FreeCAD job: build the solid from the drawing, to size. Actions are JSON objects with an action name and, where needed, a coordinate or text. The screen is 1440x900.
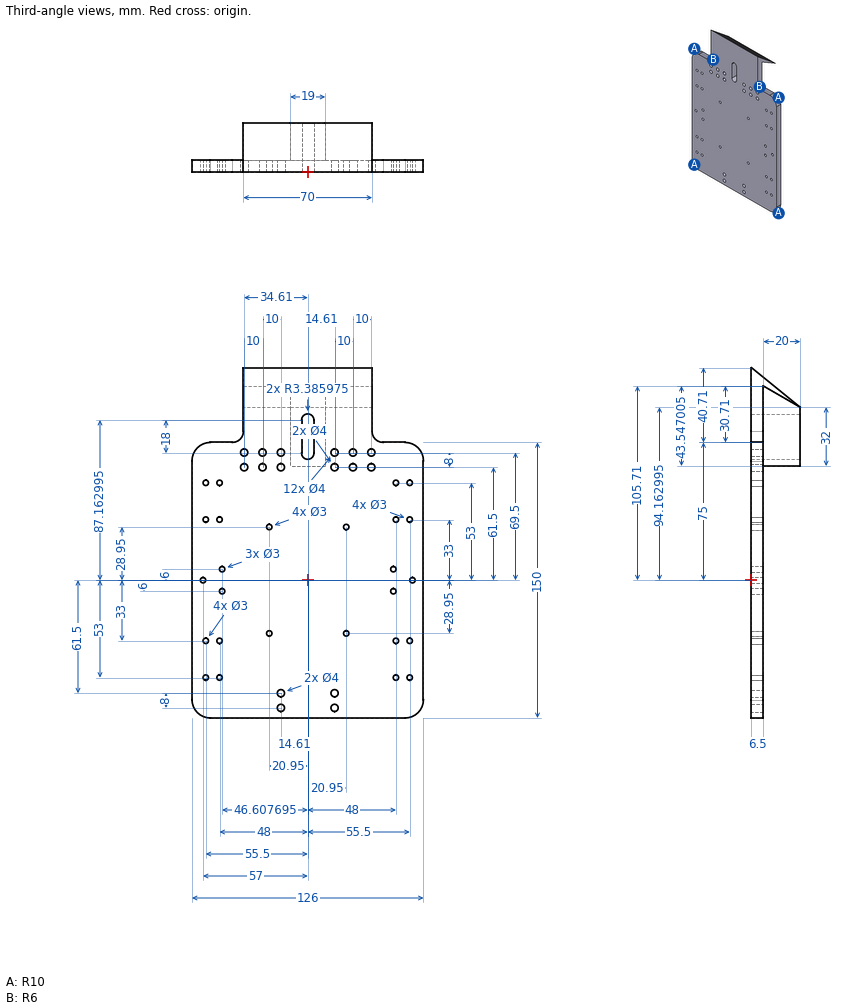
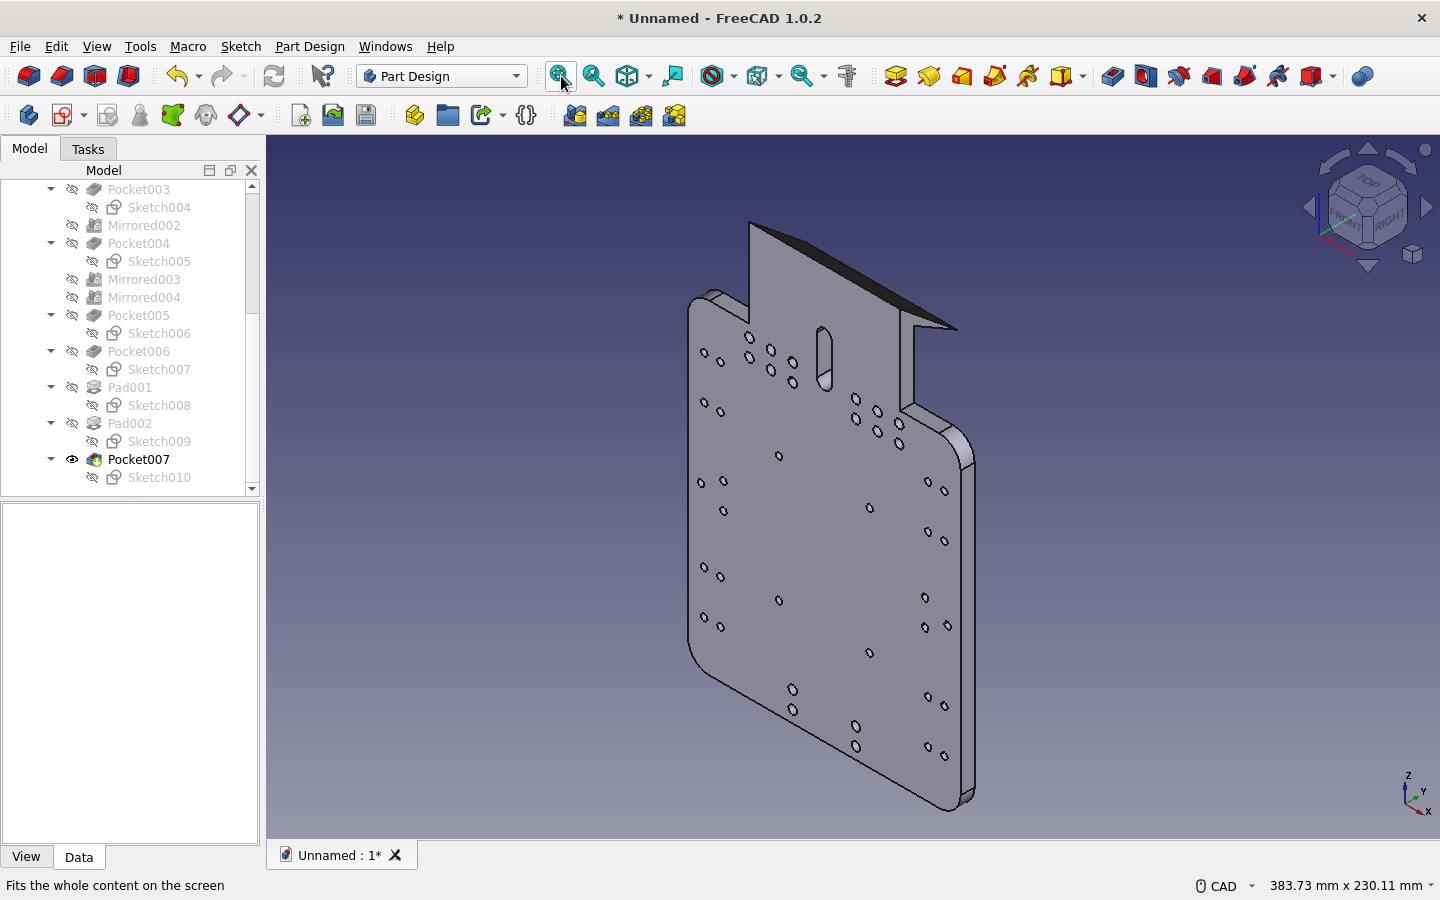
{"action": "scroll", "coordinate": [756, 318], "scroll_direction": "up", "scroll_amount": 4}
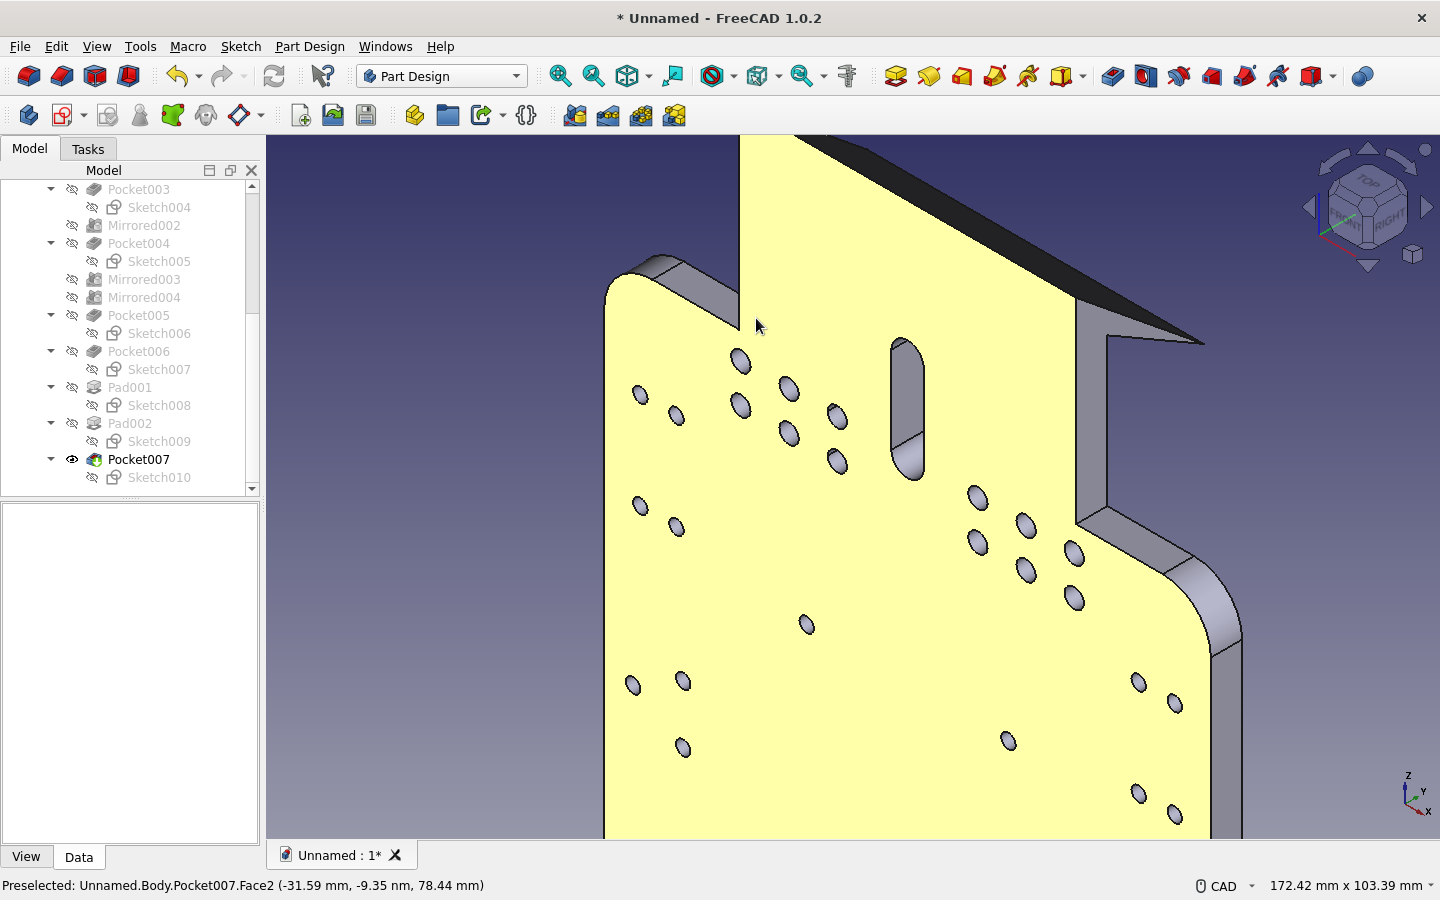
{"action": "key", "text": "v f"}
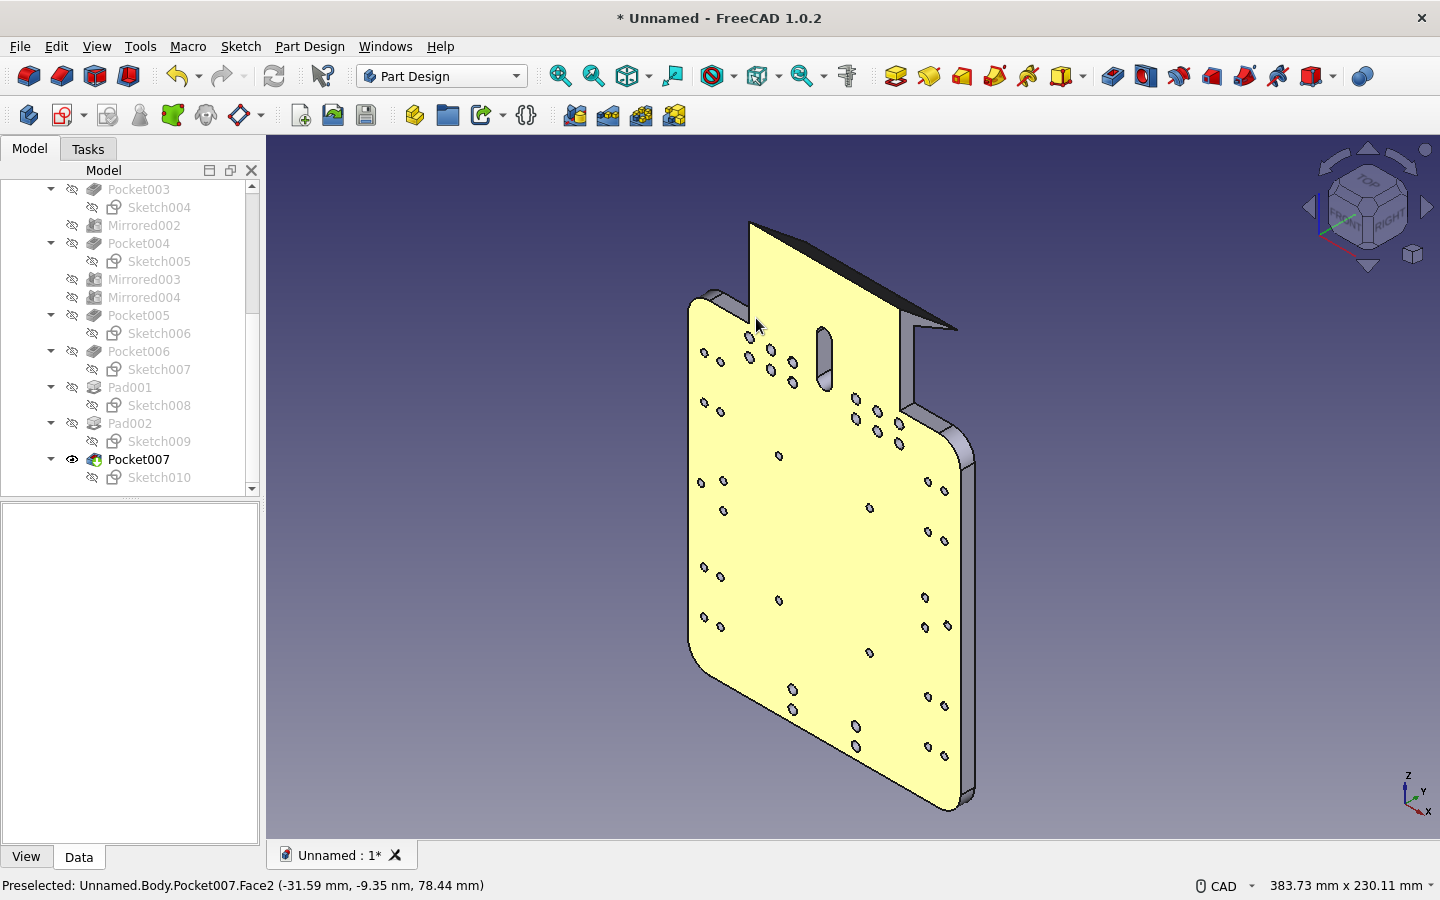
{"action": "key", "text": "2"}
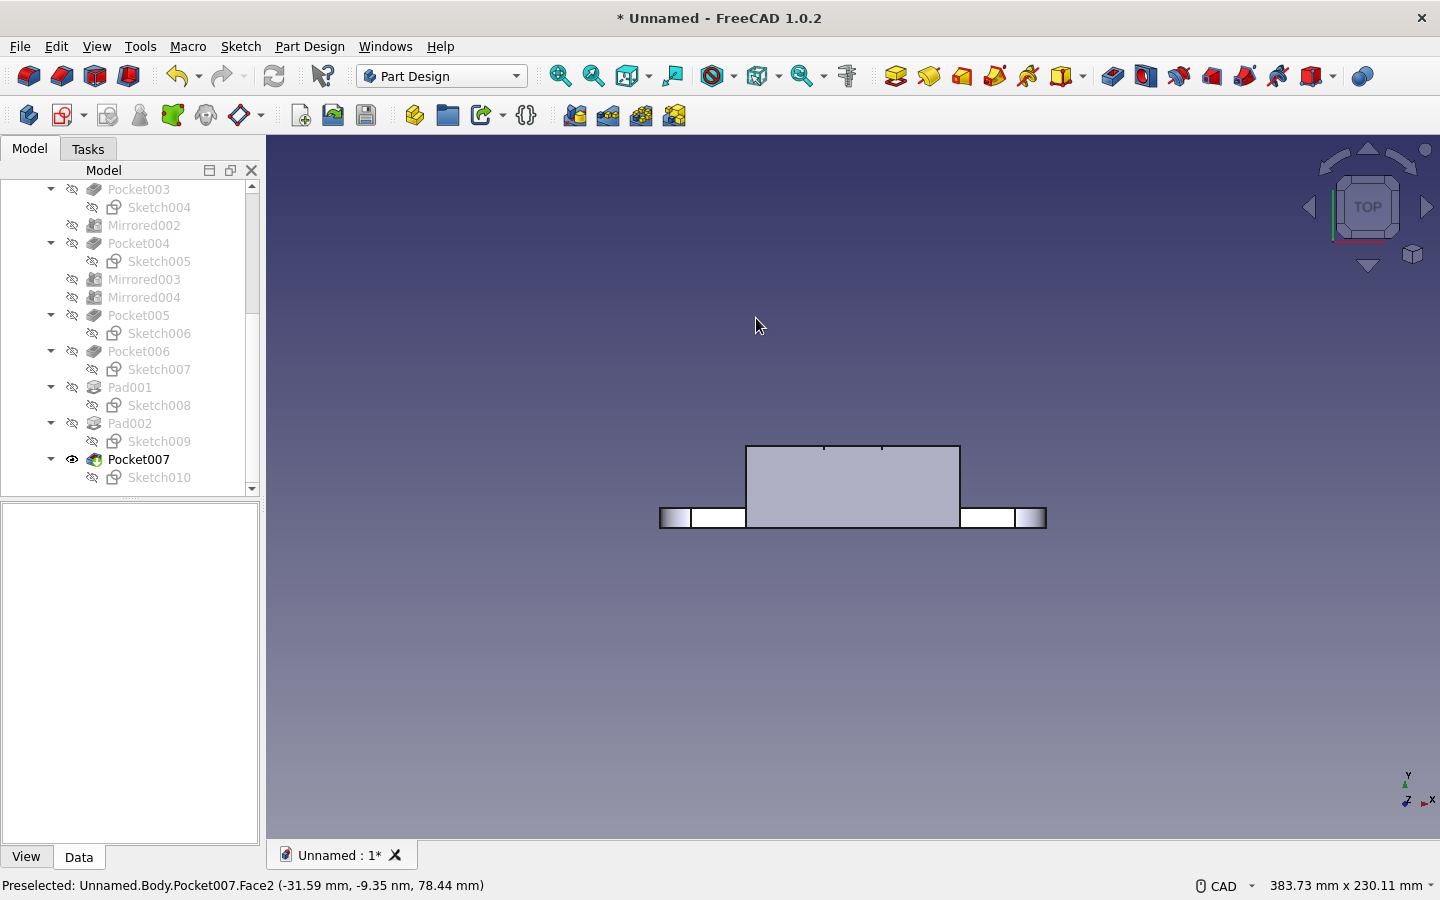
{"action": "left_click", "coordinate": [561, 76]}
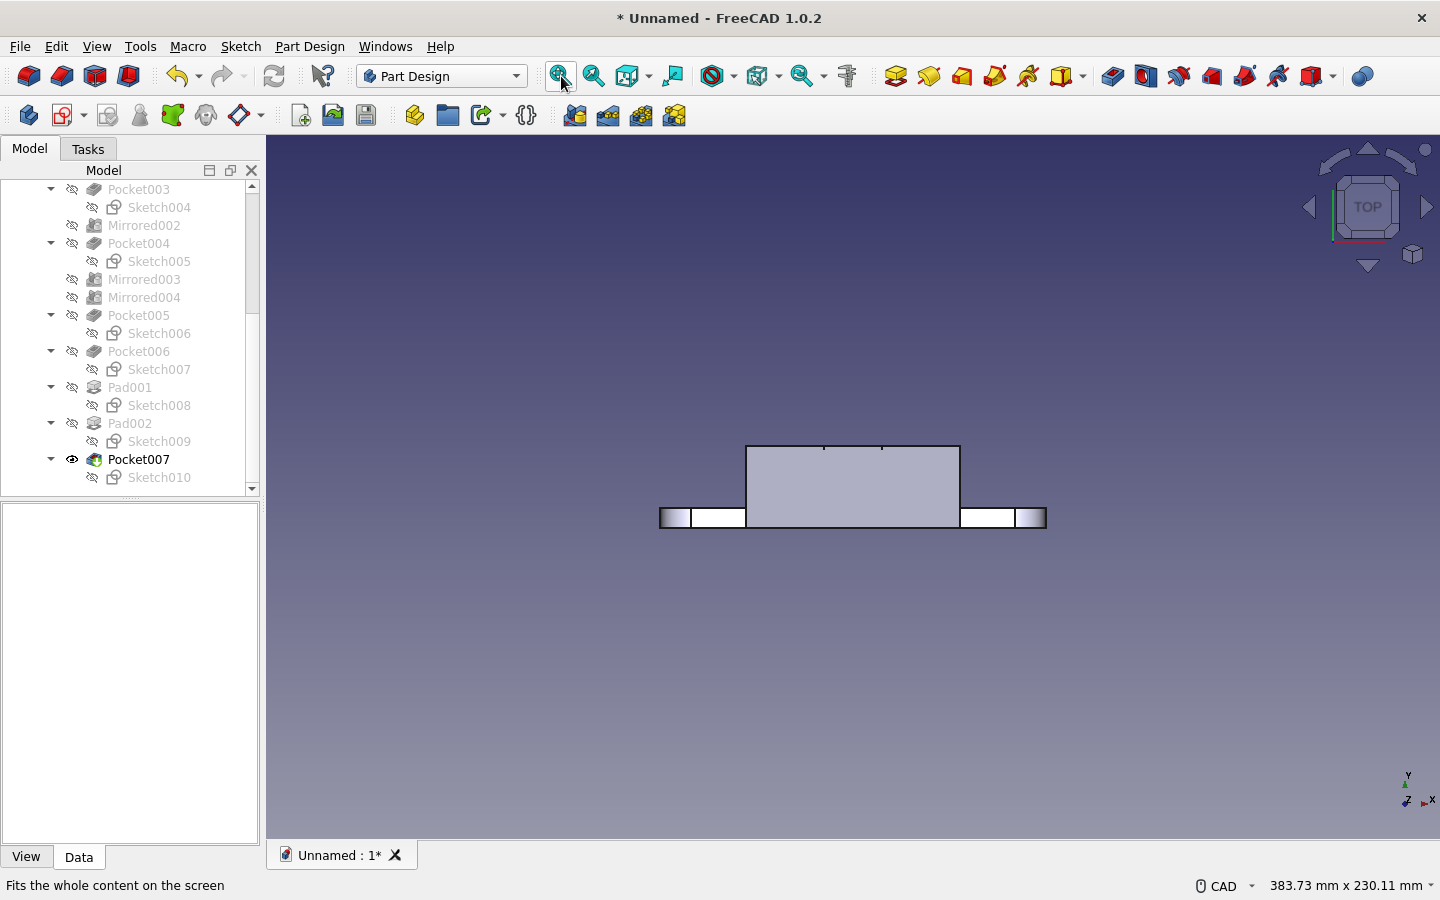
{"action": "scroll", "coordinate": [746, 517], "scroll_direction": "up", "scroll_amount": 4}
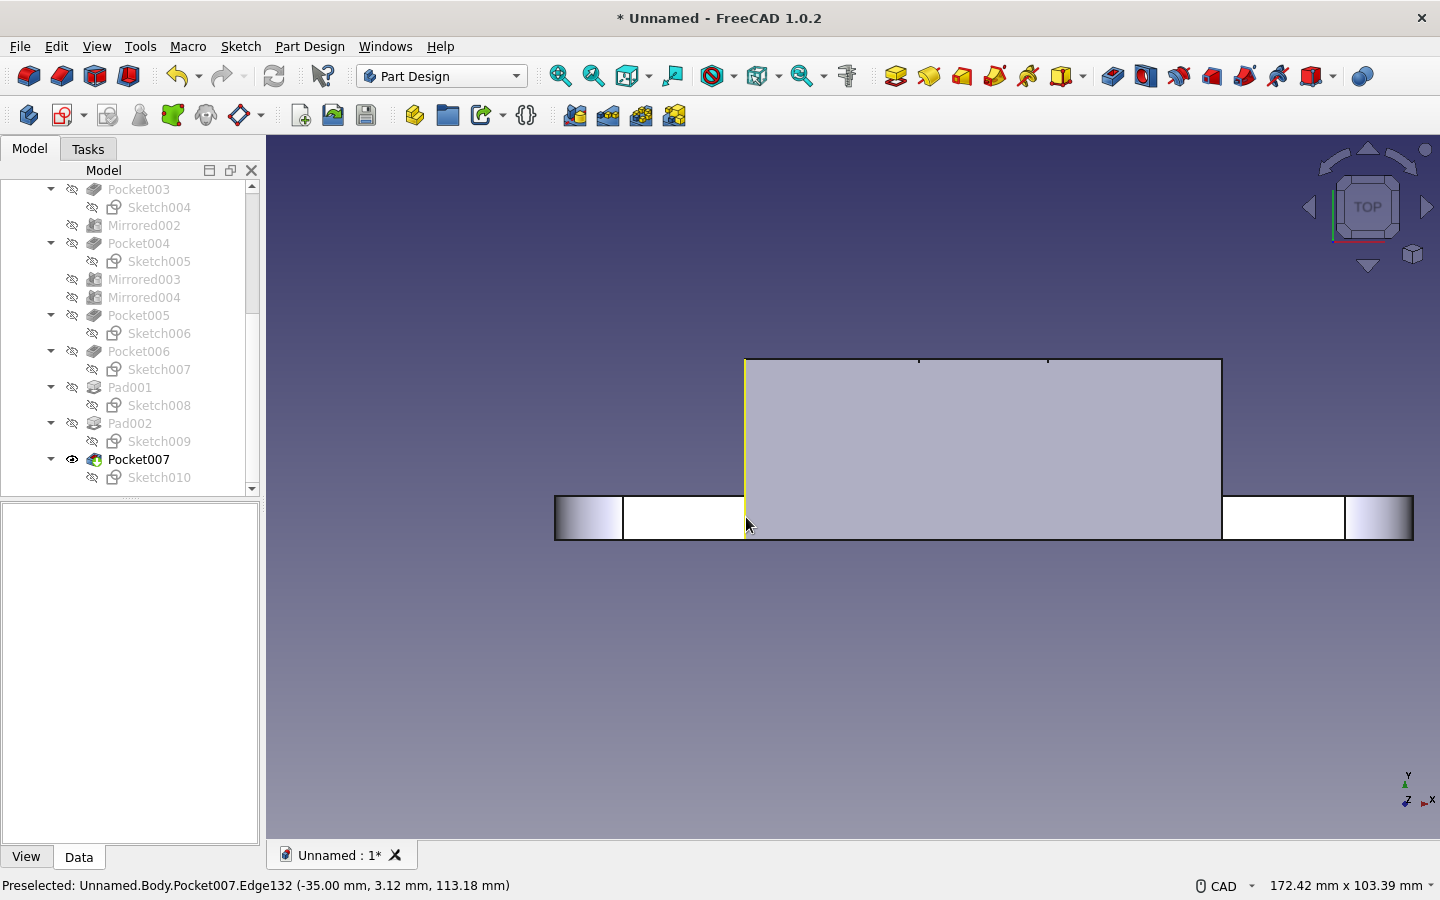
{"action": "left_click", "coordinate": [561, 76]}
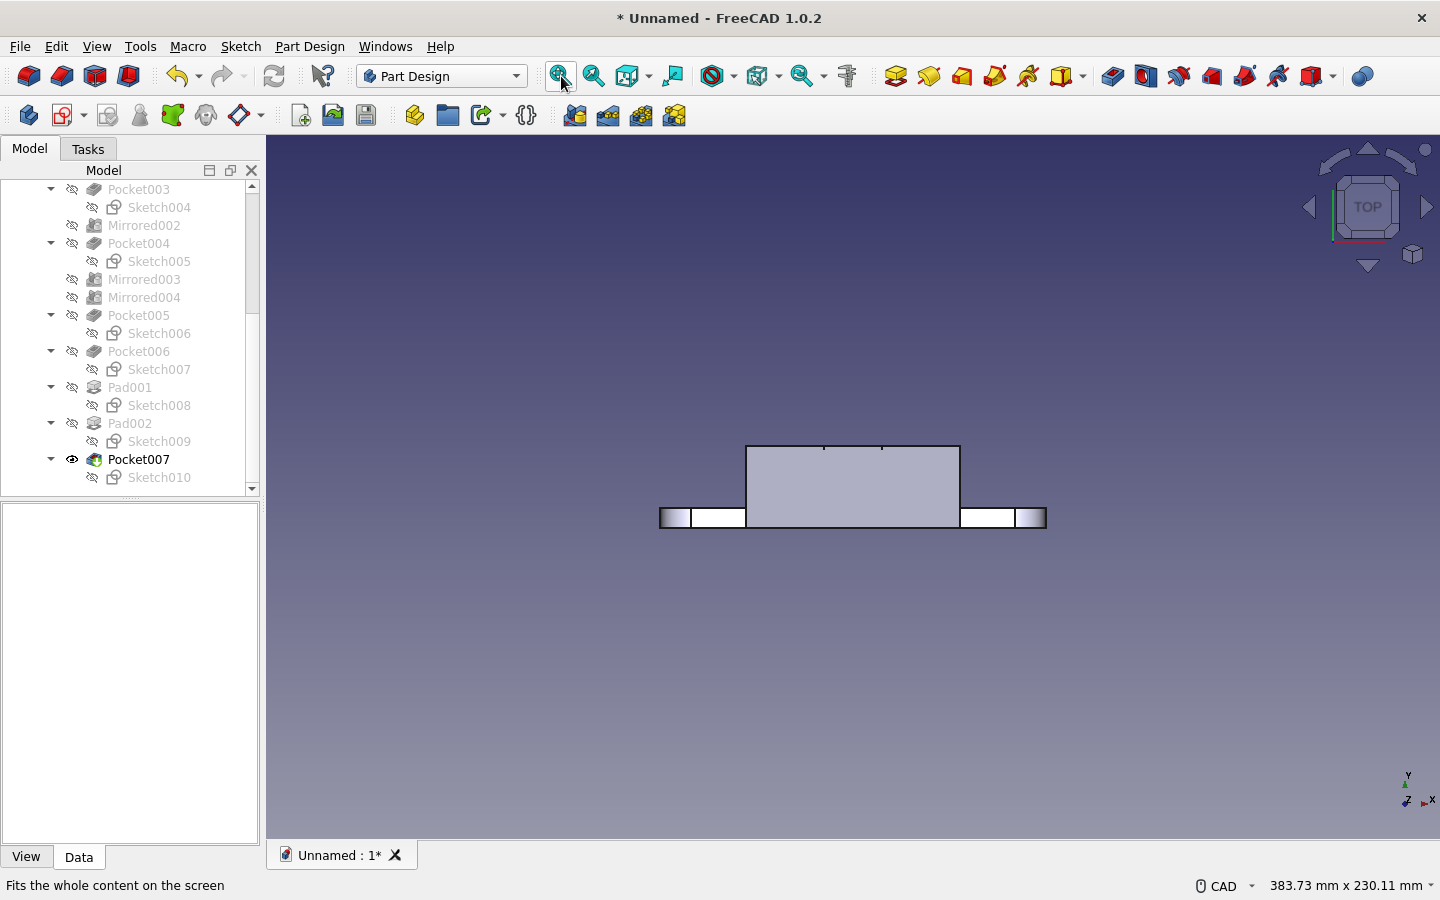
{"action": "key", "text": "1"}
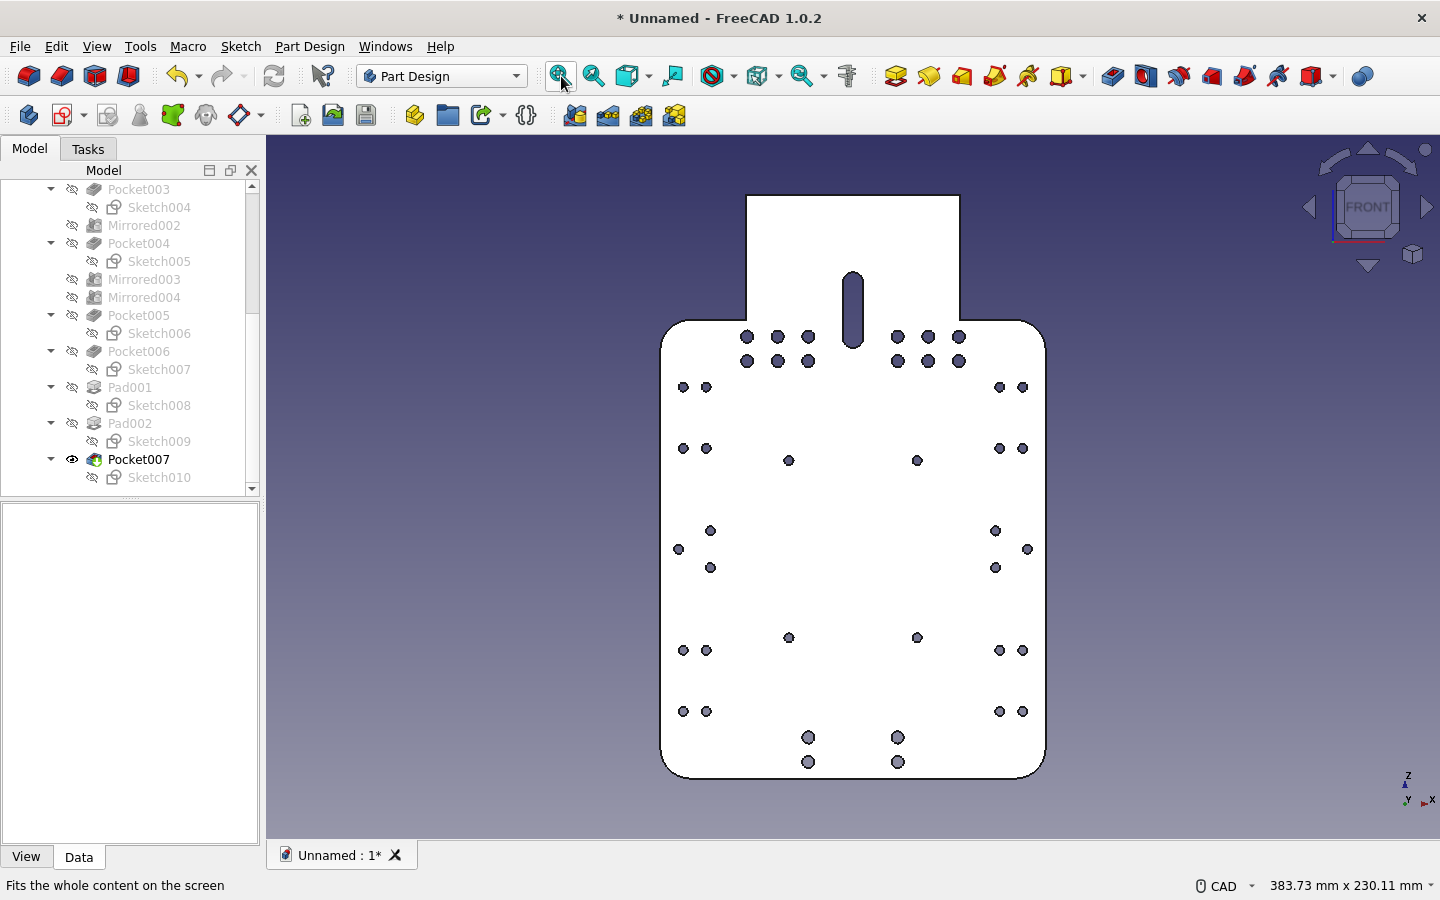
{"action": "scroll", "coordinate": [746, 319], "scroll_direction": "up", "scroll_amount": 4}